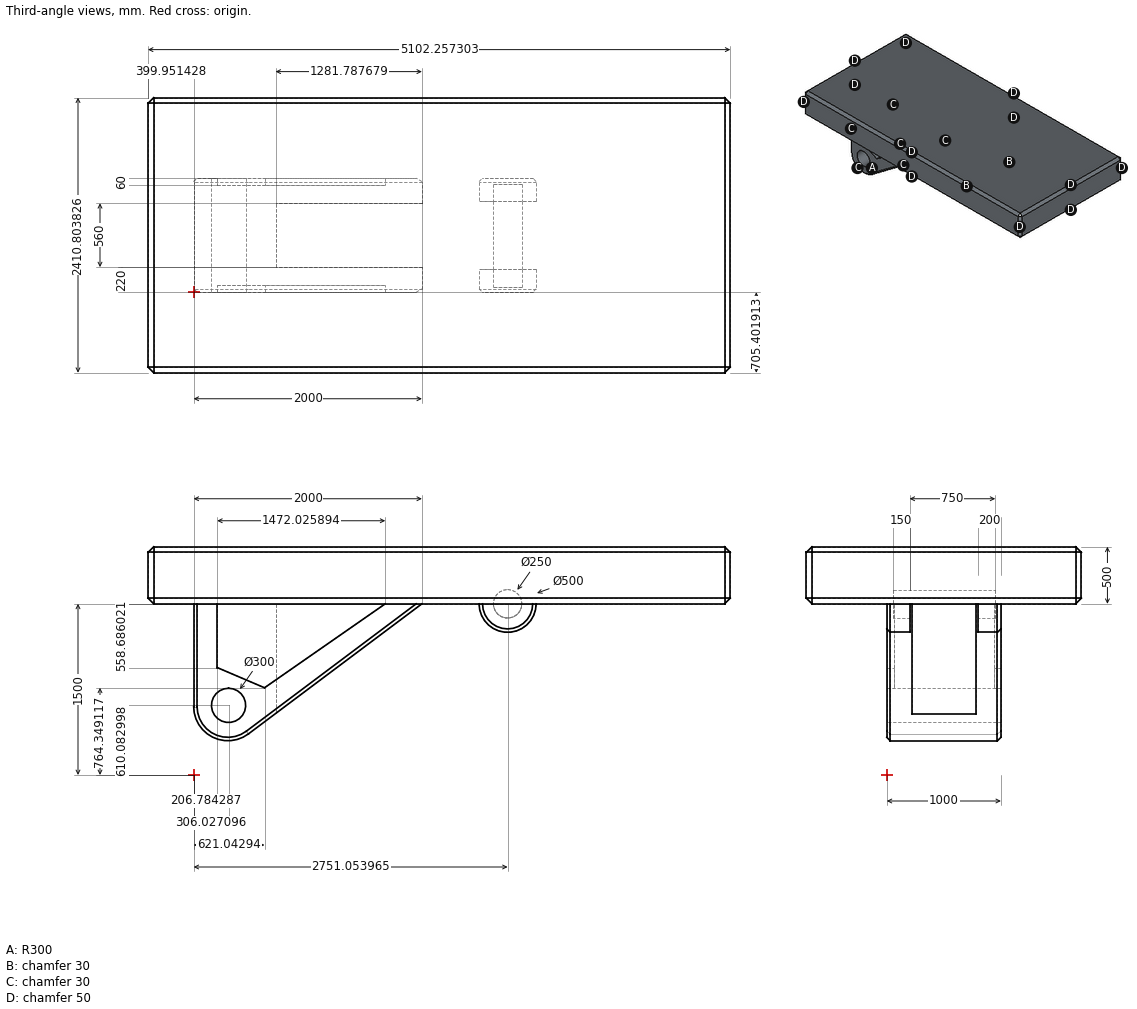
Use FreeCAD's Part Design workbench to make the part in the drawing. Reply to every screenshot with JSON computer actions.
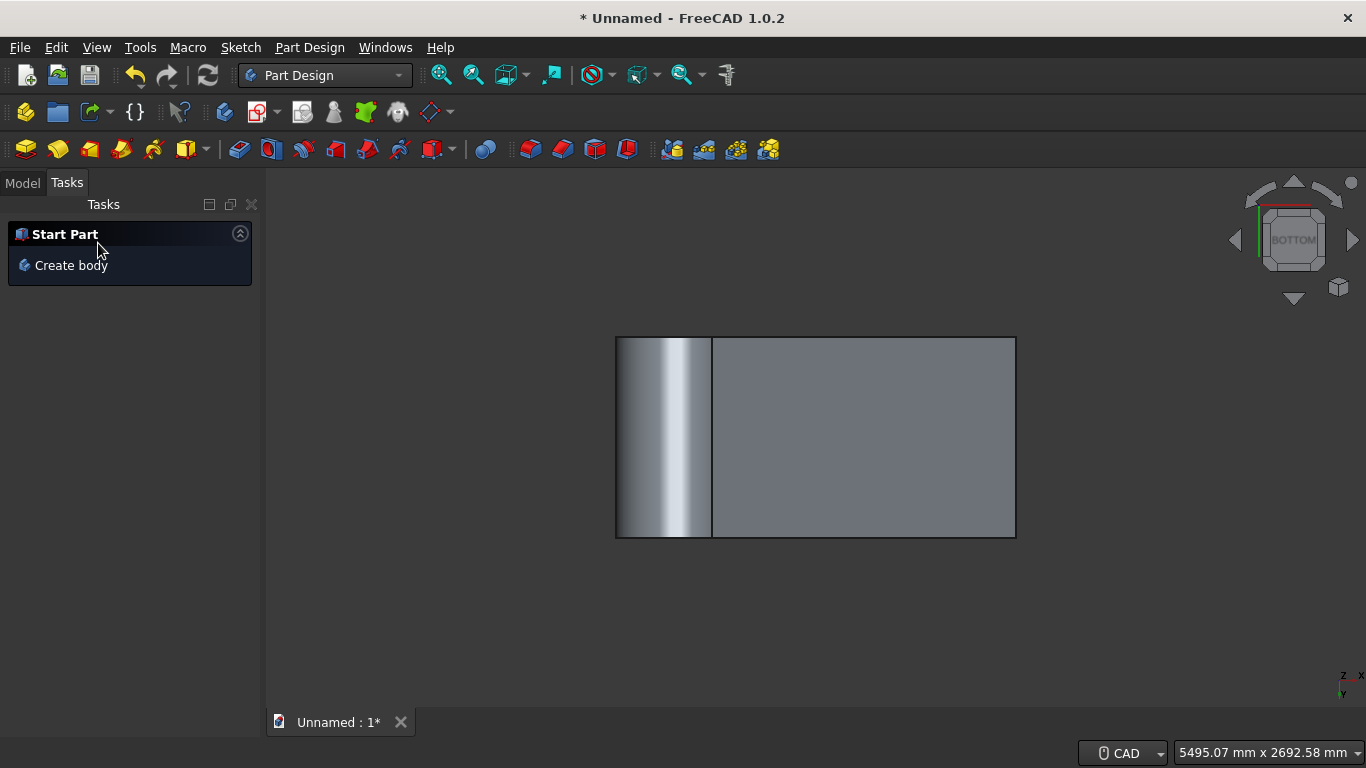
{"action": "left_click", "coordinate": [442, 76]}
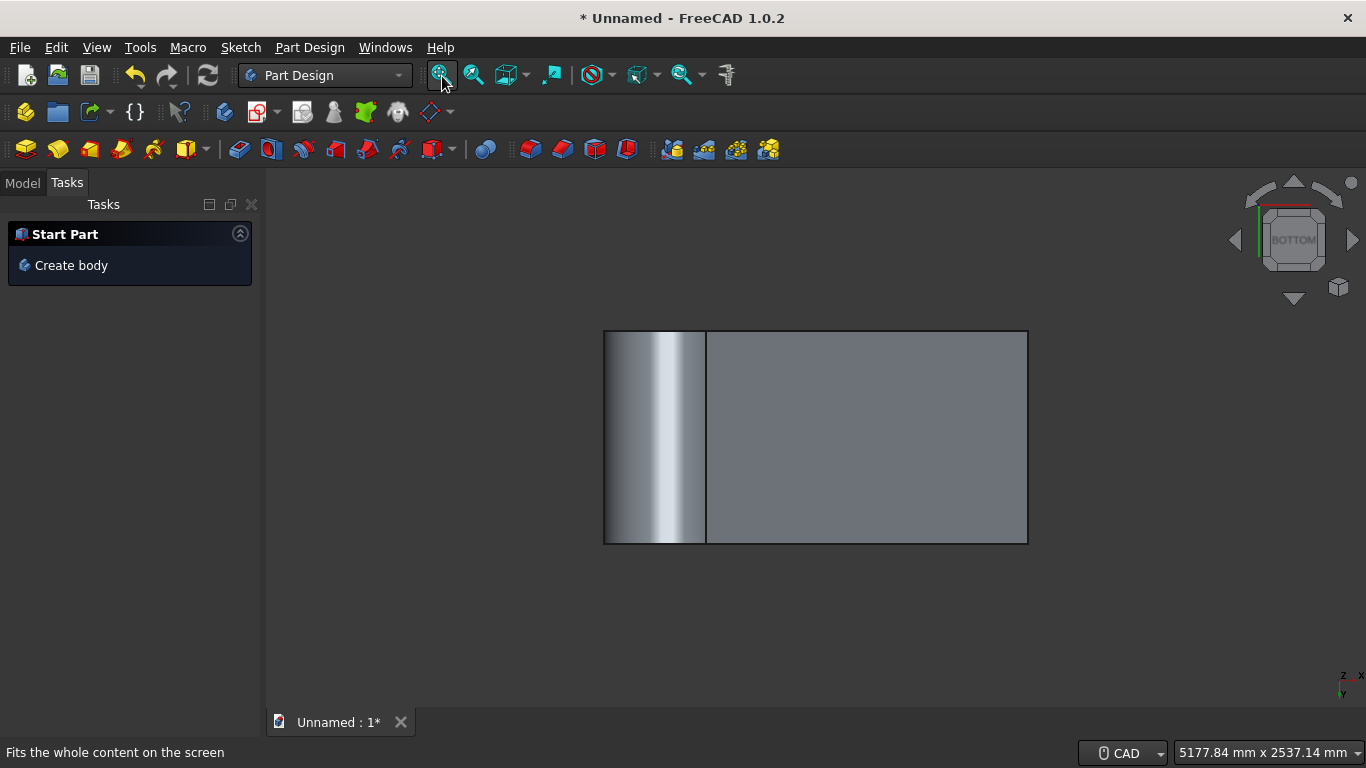
{"action": "key", "text": "0"}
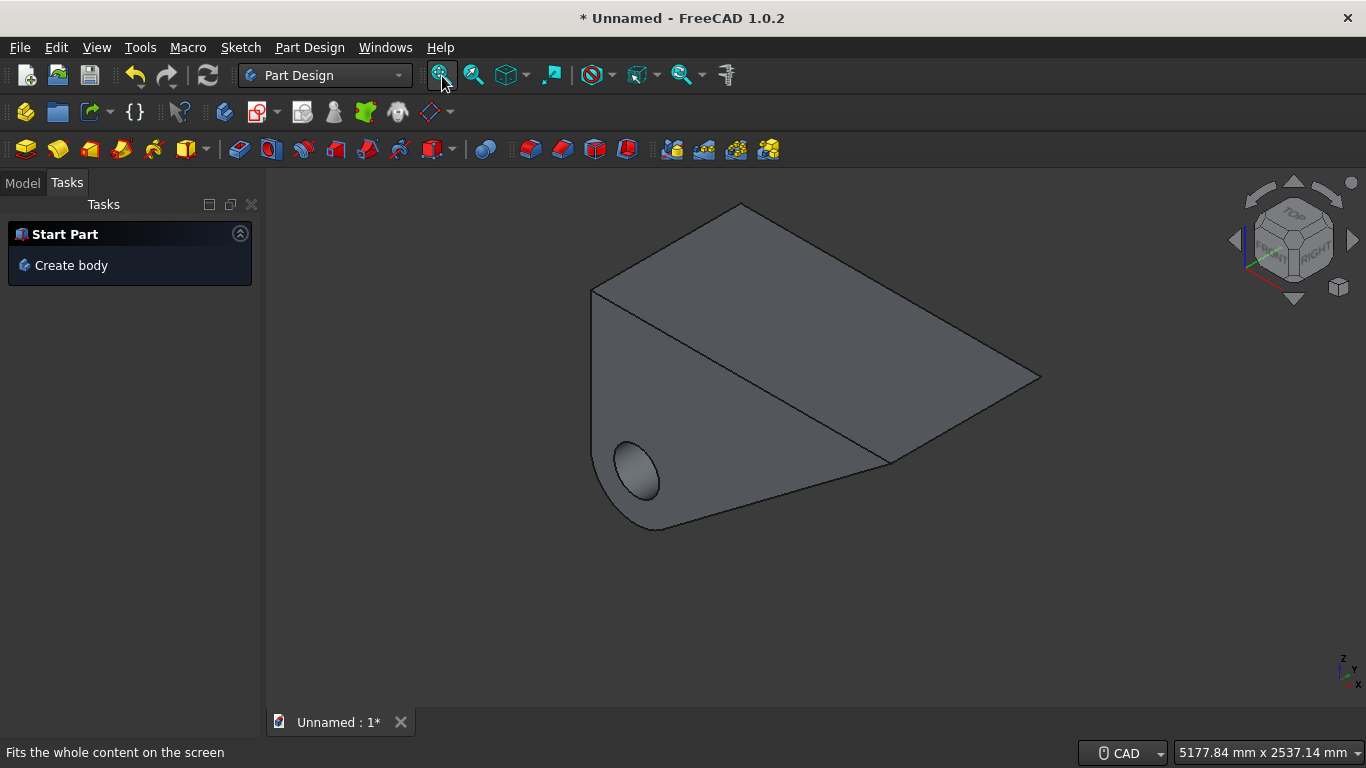
{"action": "left_click", "coordinate": [859, 357]}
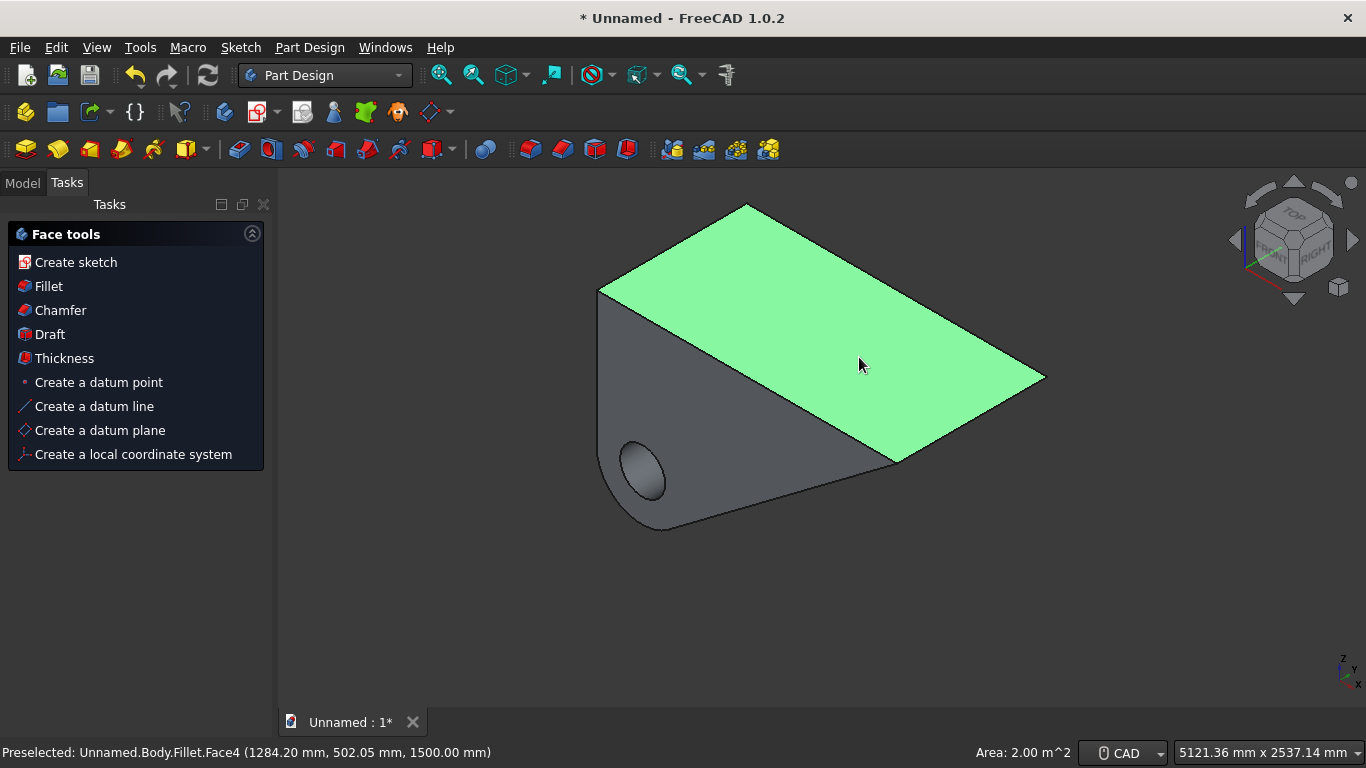
{"action": "left_click", "coordinate": [258, 112]}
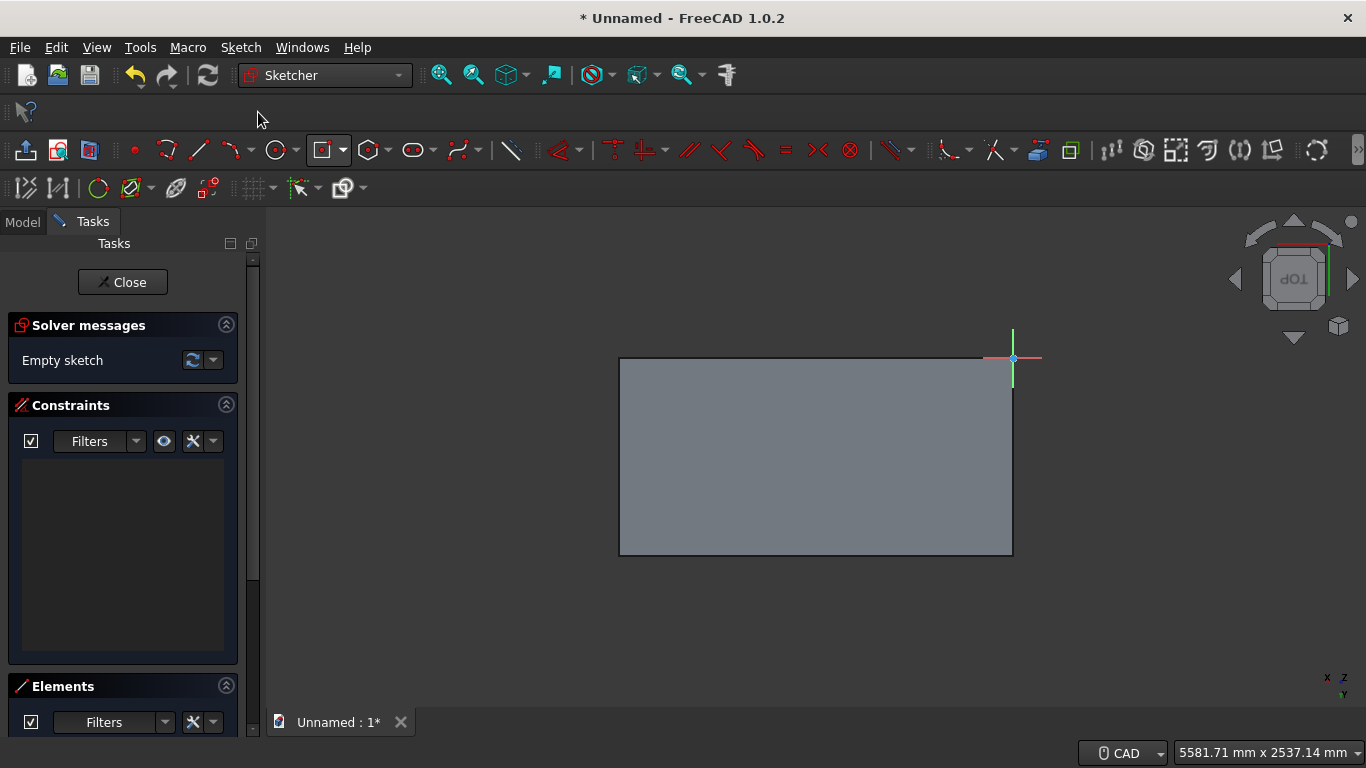
{"action": "scroll", "coordinate": [1069, 457], "scroll_direction": "down", "scroll_amount": 2}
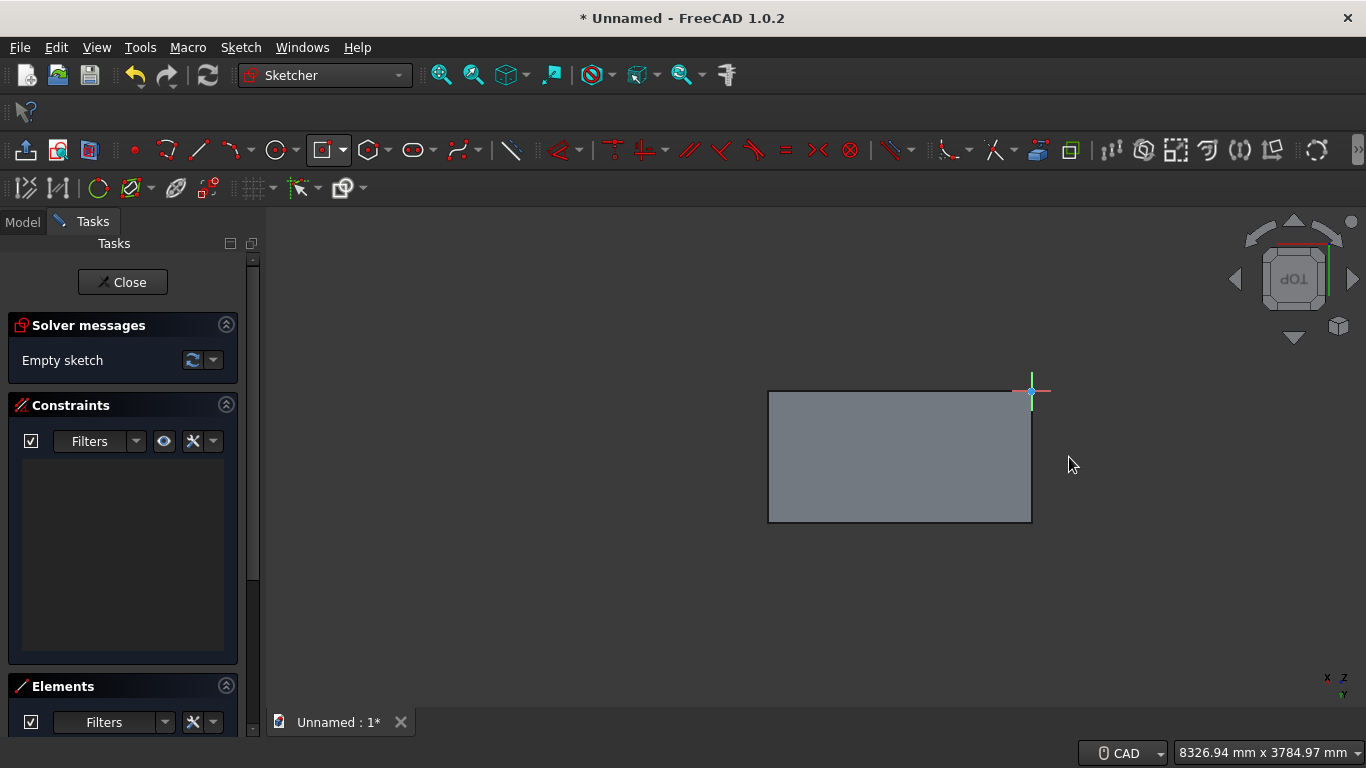
{"action": "left_click", "coordinate": [346, 150]}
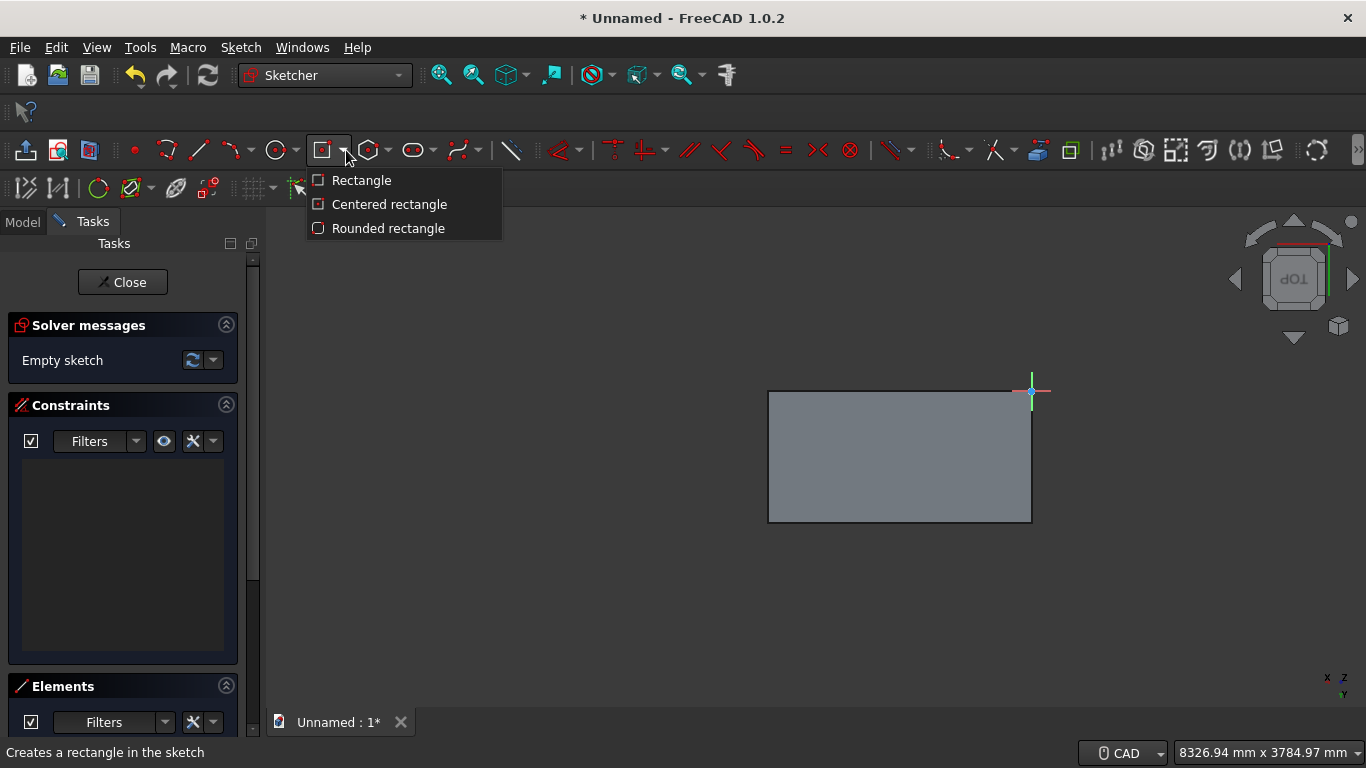
{"action": "left_click", "coordinate": [404, 180]}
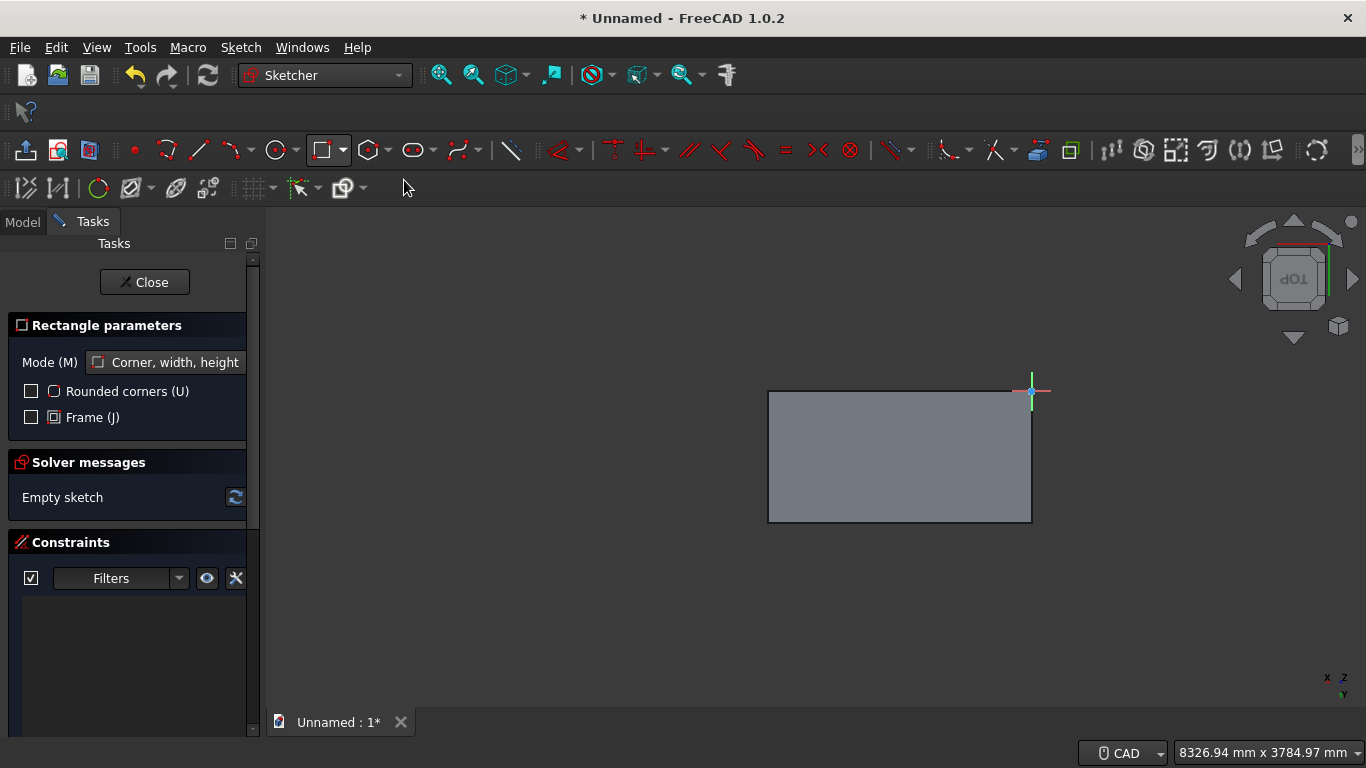
{"action": "left_click", "coordinate": [411, 298]}
{"action": "mouse_move", "coordinate": [1085, 616]}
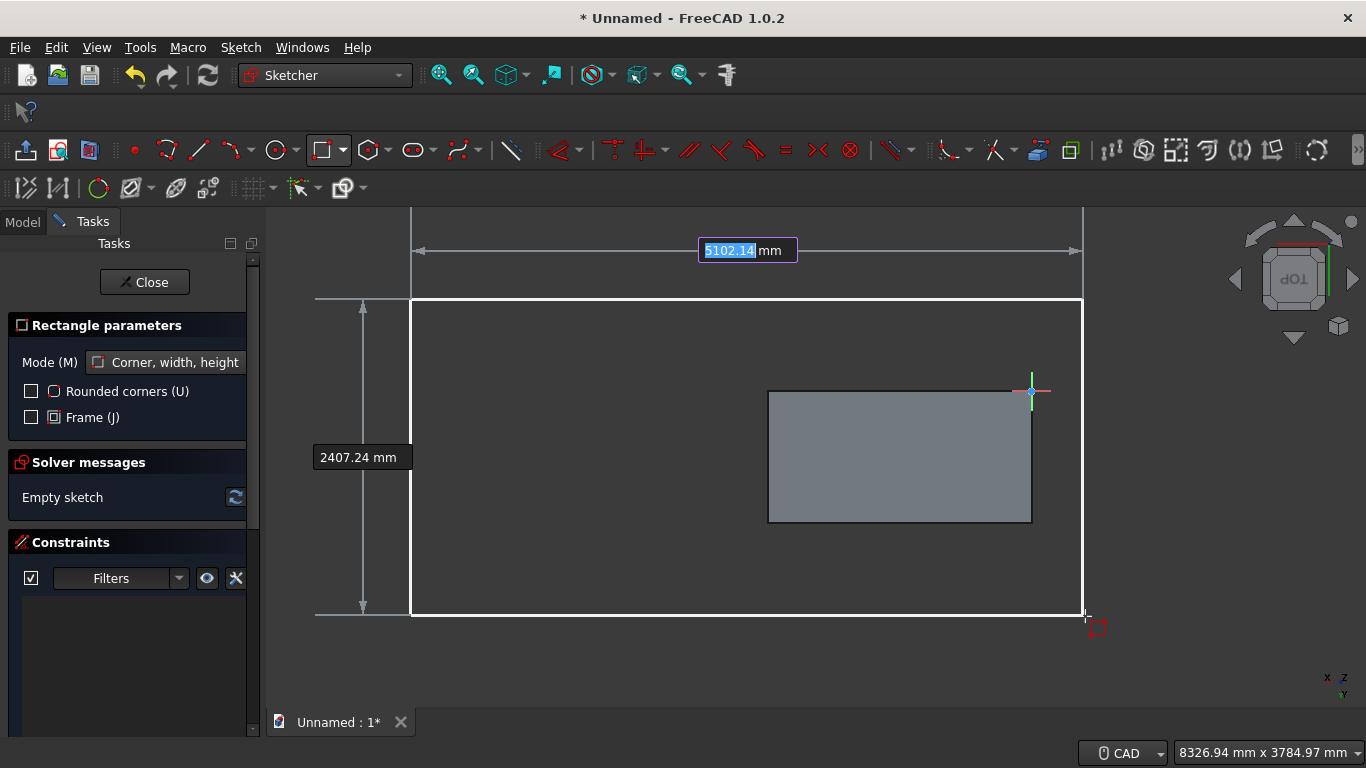
{"action": "type", "text": "5102.257303"}
{"action": "key", "text": "Tab"}
{"action": "type", "text": "2410.803826"}
{"action": "key", "text": "Return"}
{"action": "key", "text": "Escape"}